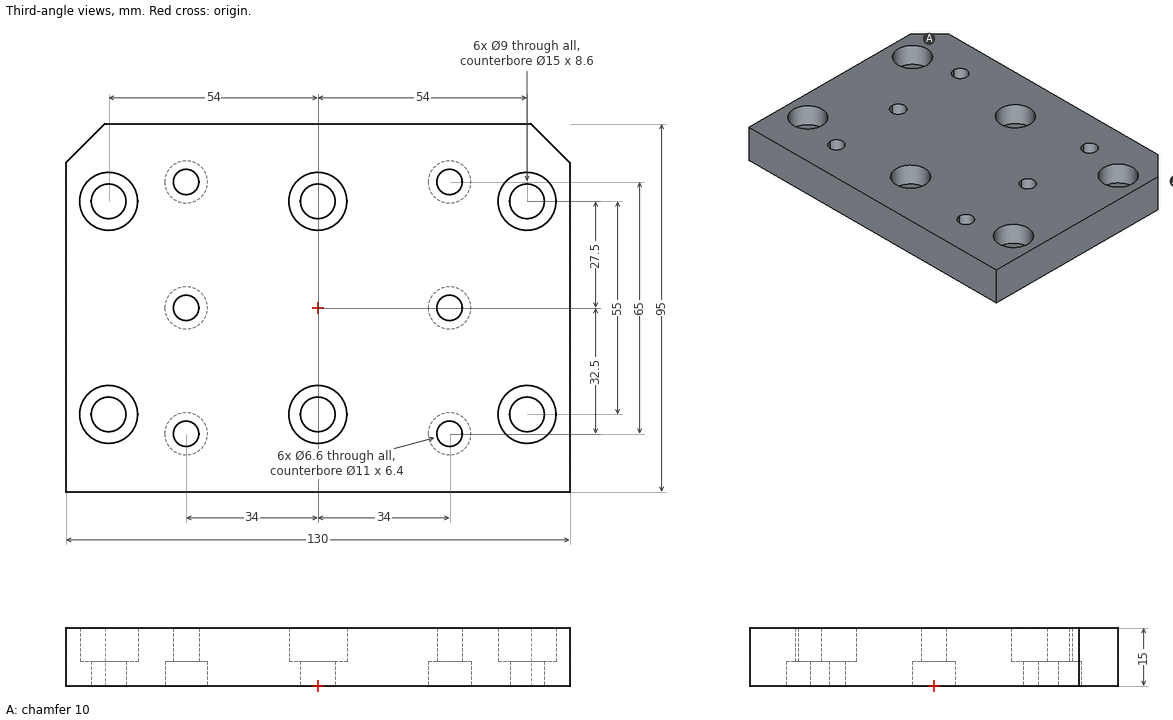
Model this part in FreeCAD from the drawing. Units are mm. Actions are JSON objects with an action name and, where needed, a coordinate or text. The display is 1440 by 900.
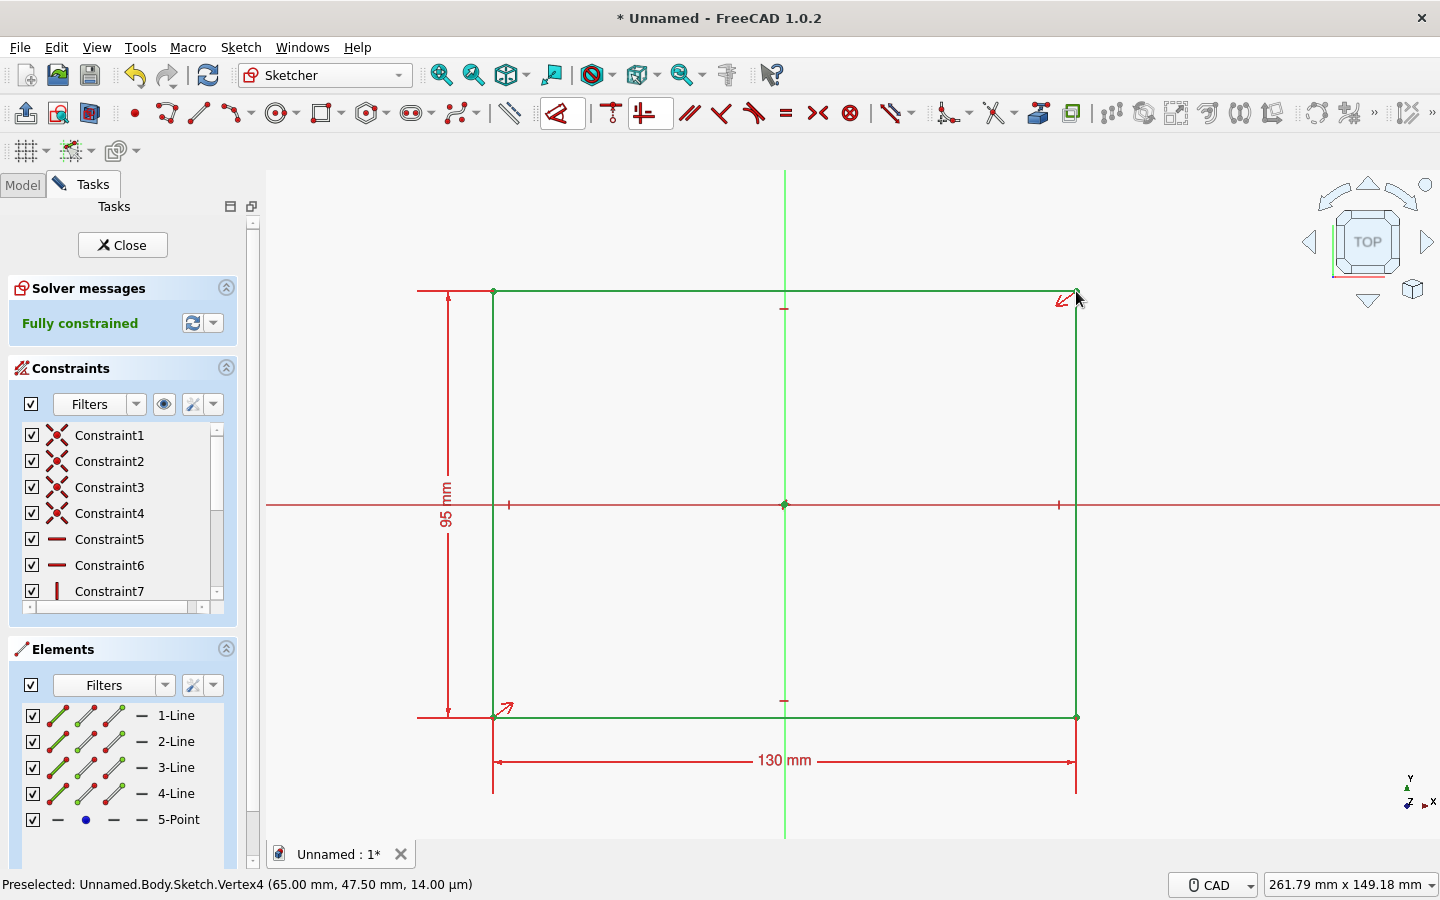
{"action": "left_click", "coordinate": [123, 245]}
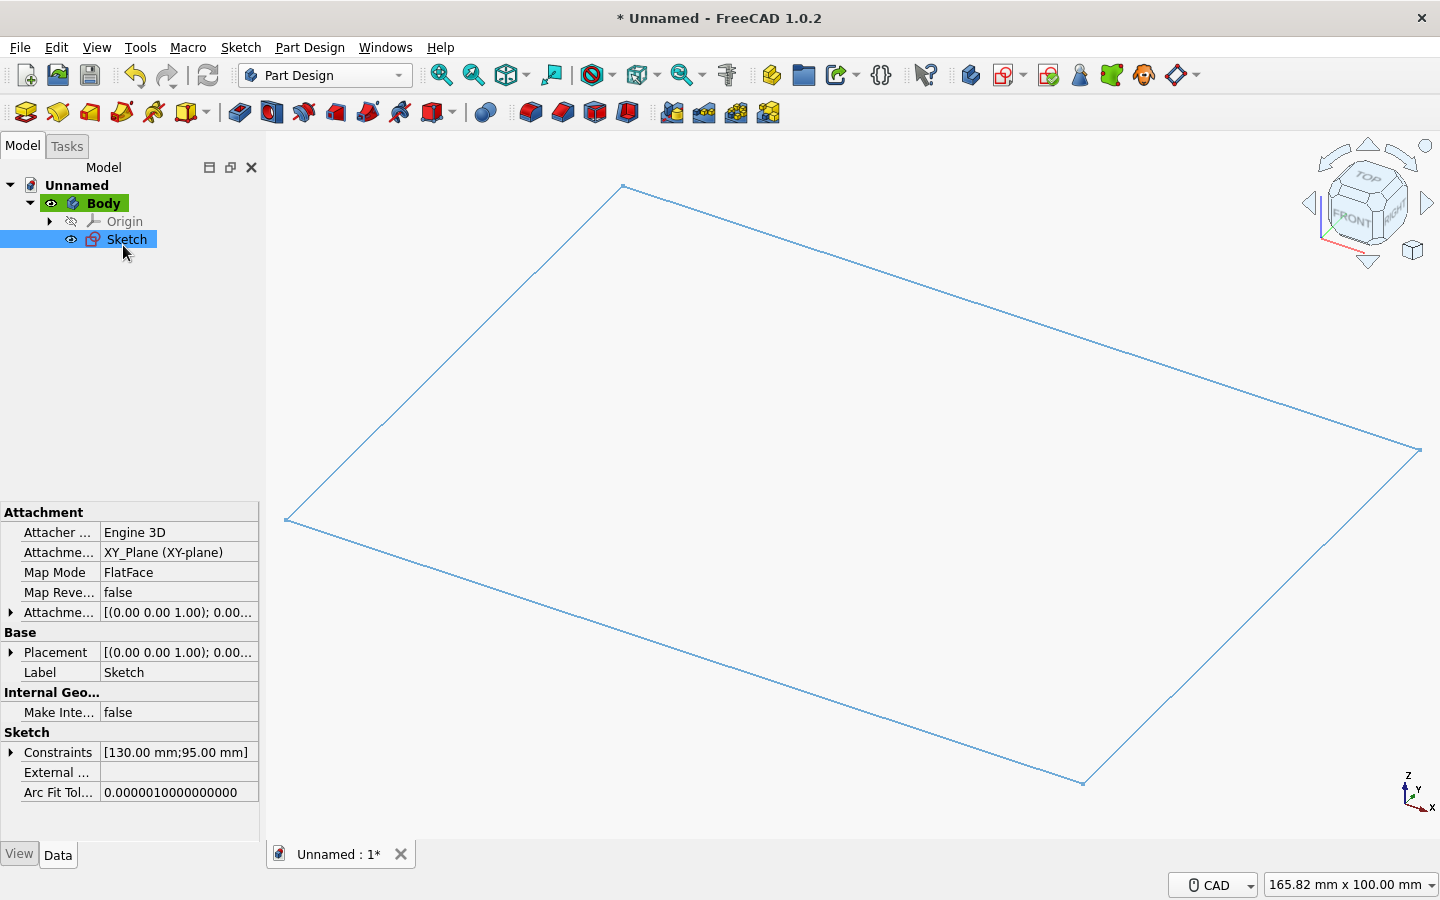
{"action": "left_click", "coordinate": [26, 112]}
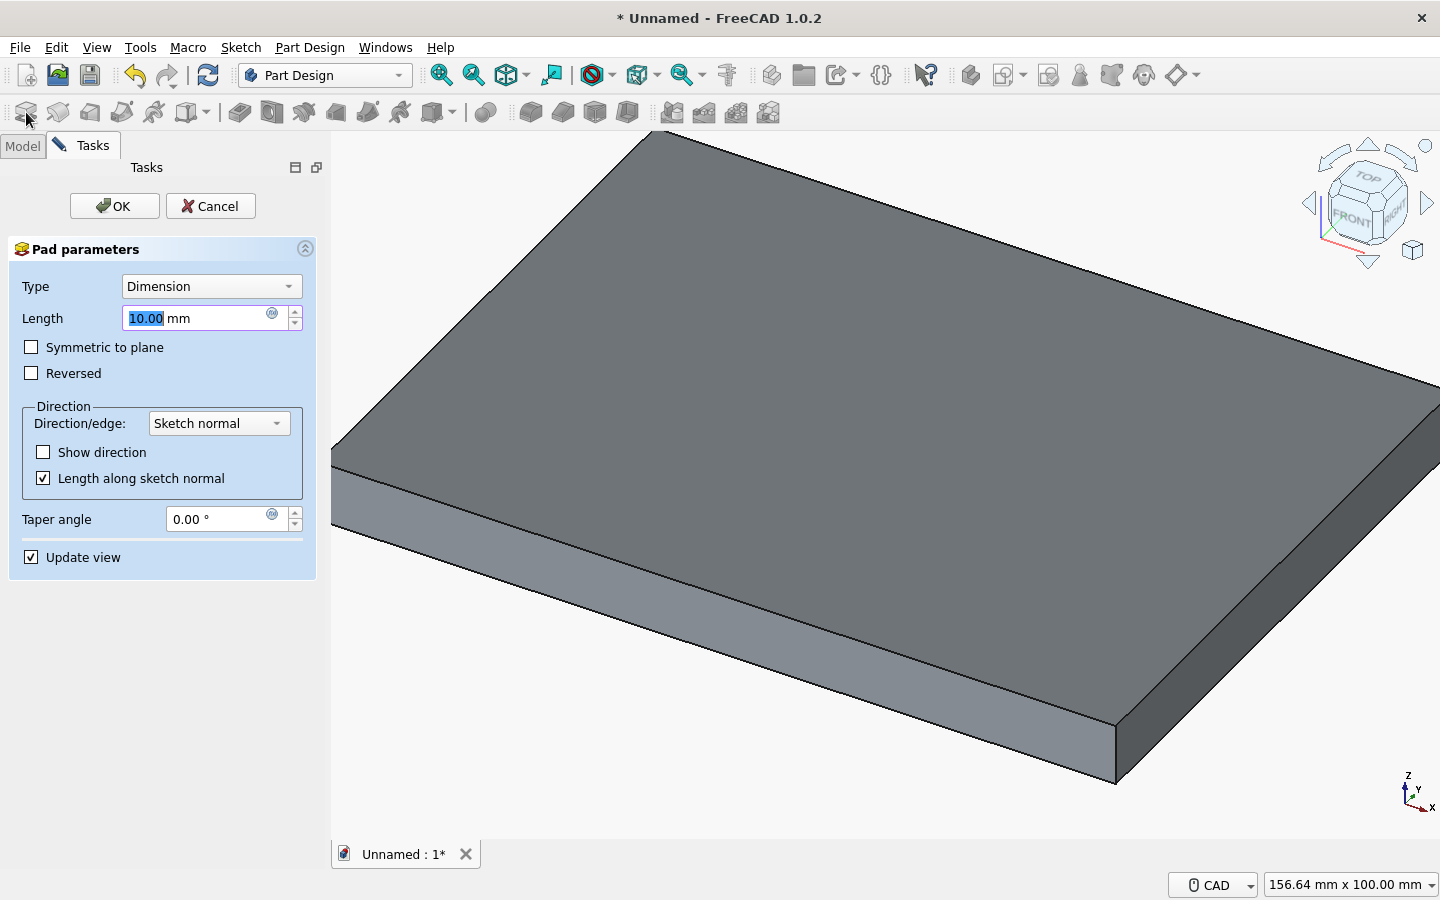
{"action": "type", "text": "15"}
{"action": "key", "text": "Tab"}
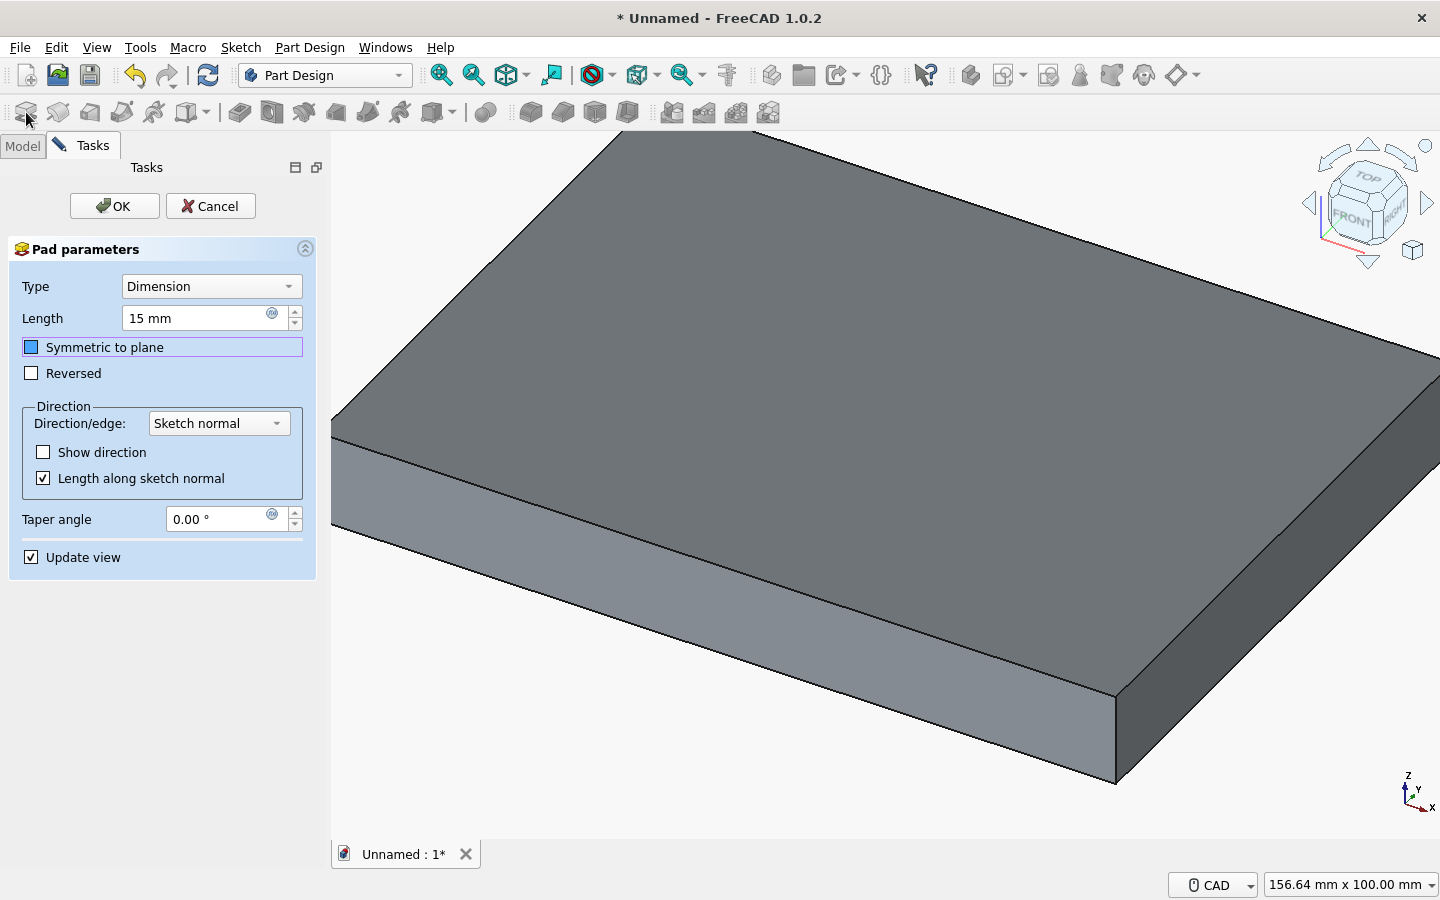
{"action": "left_click", "coordinate": [115, 206]}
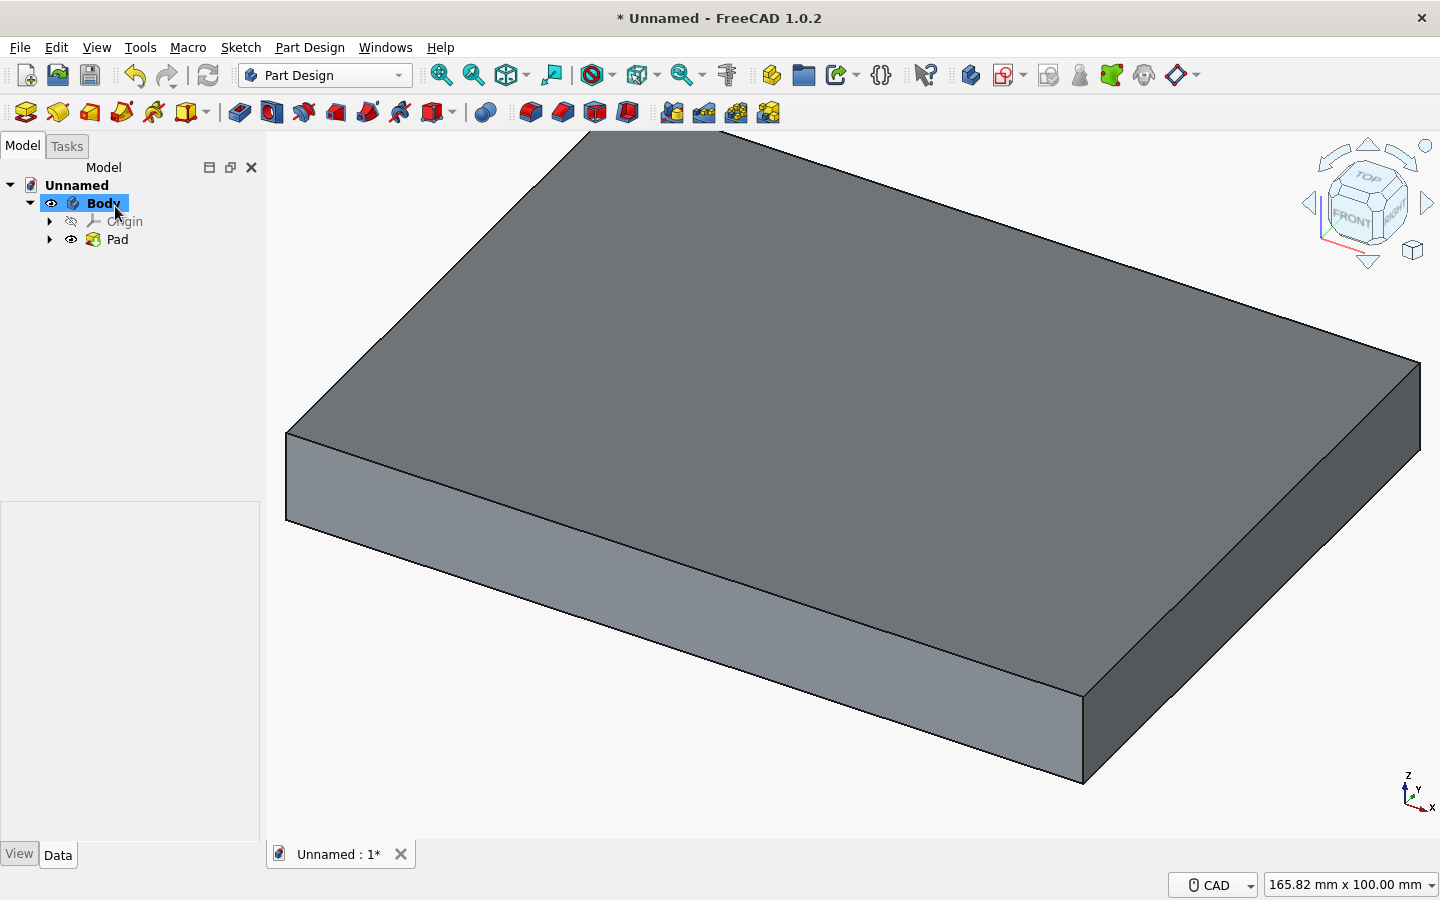
{"action": "key", "text": "v f"}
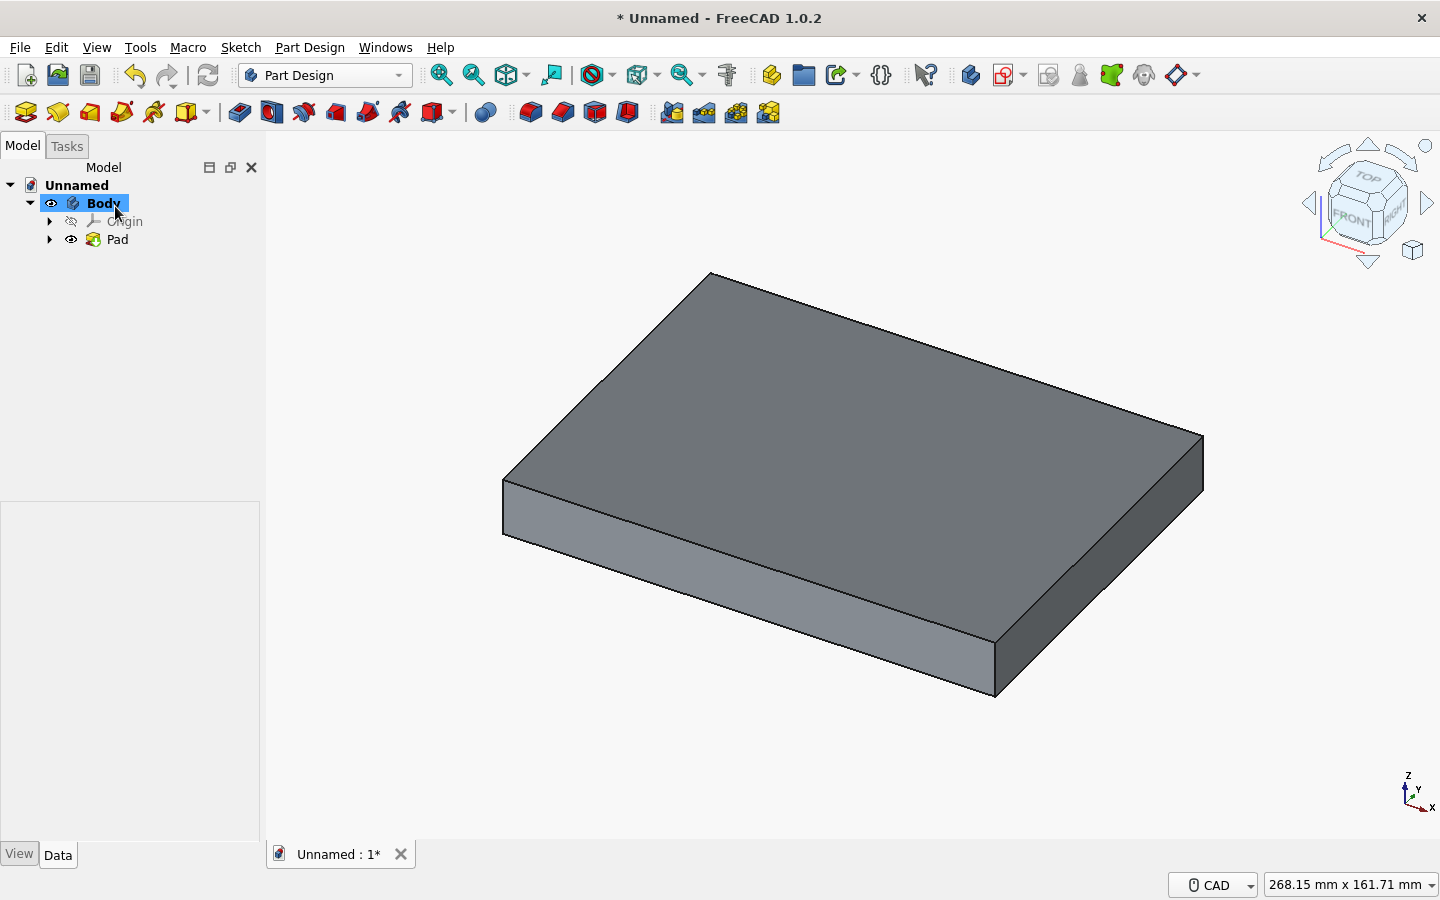
{"action": "left_click", "coordinate": [853, 457]}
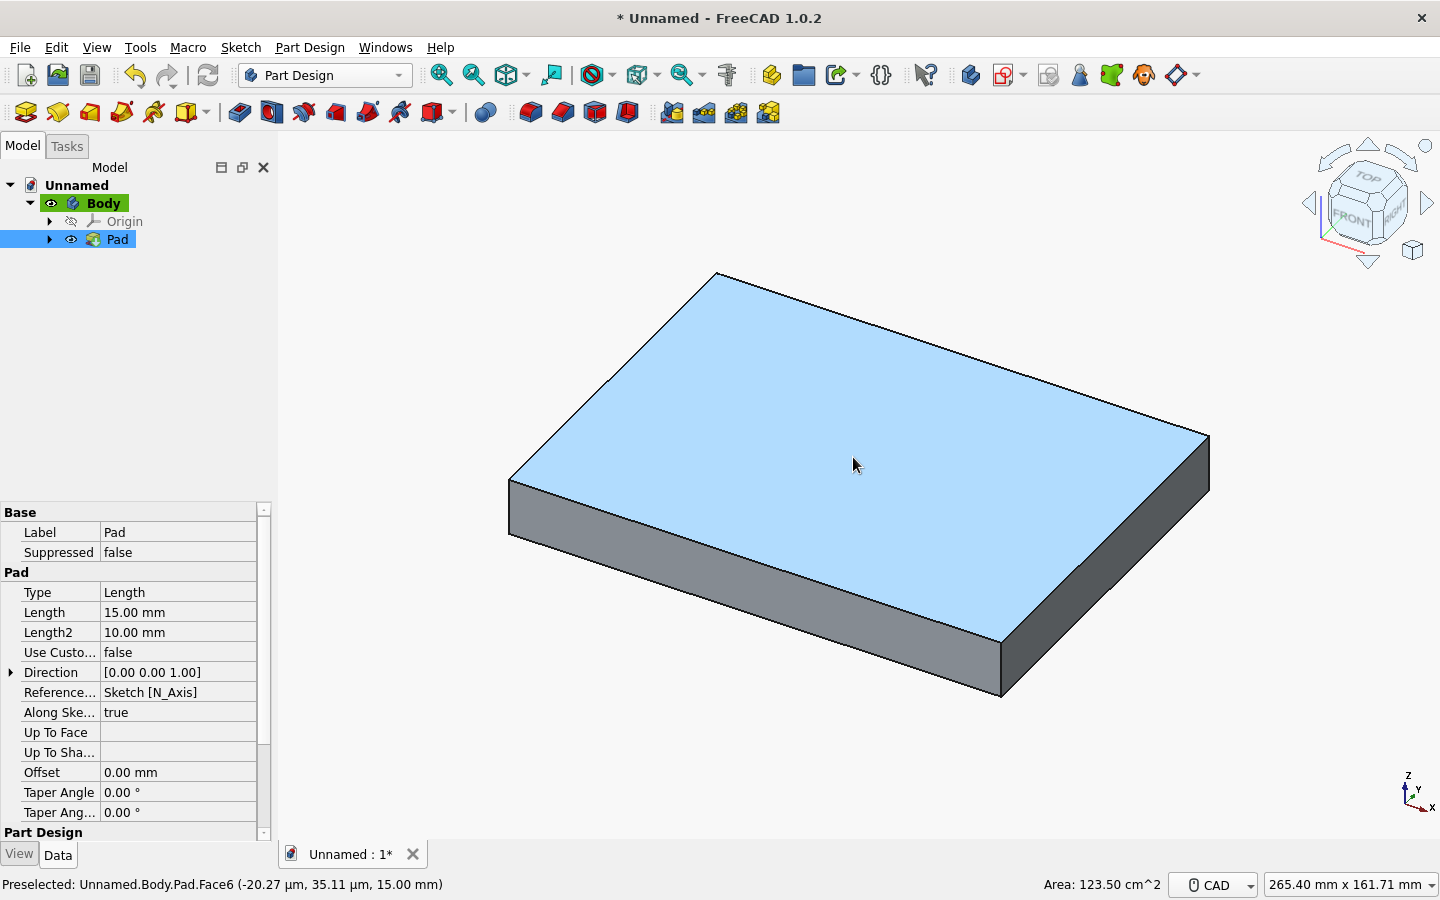
{"action": "left_click", "coordinate": [1004, 76]}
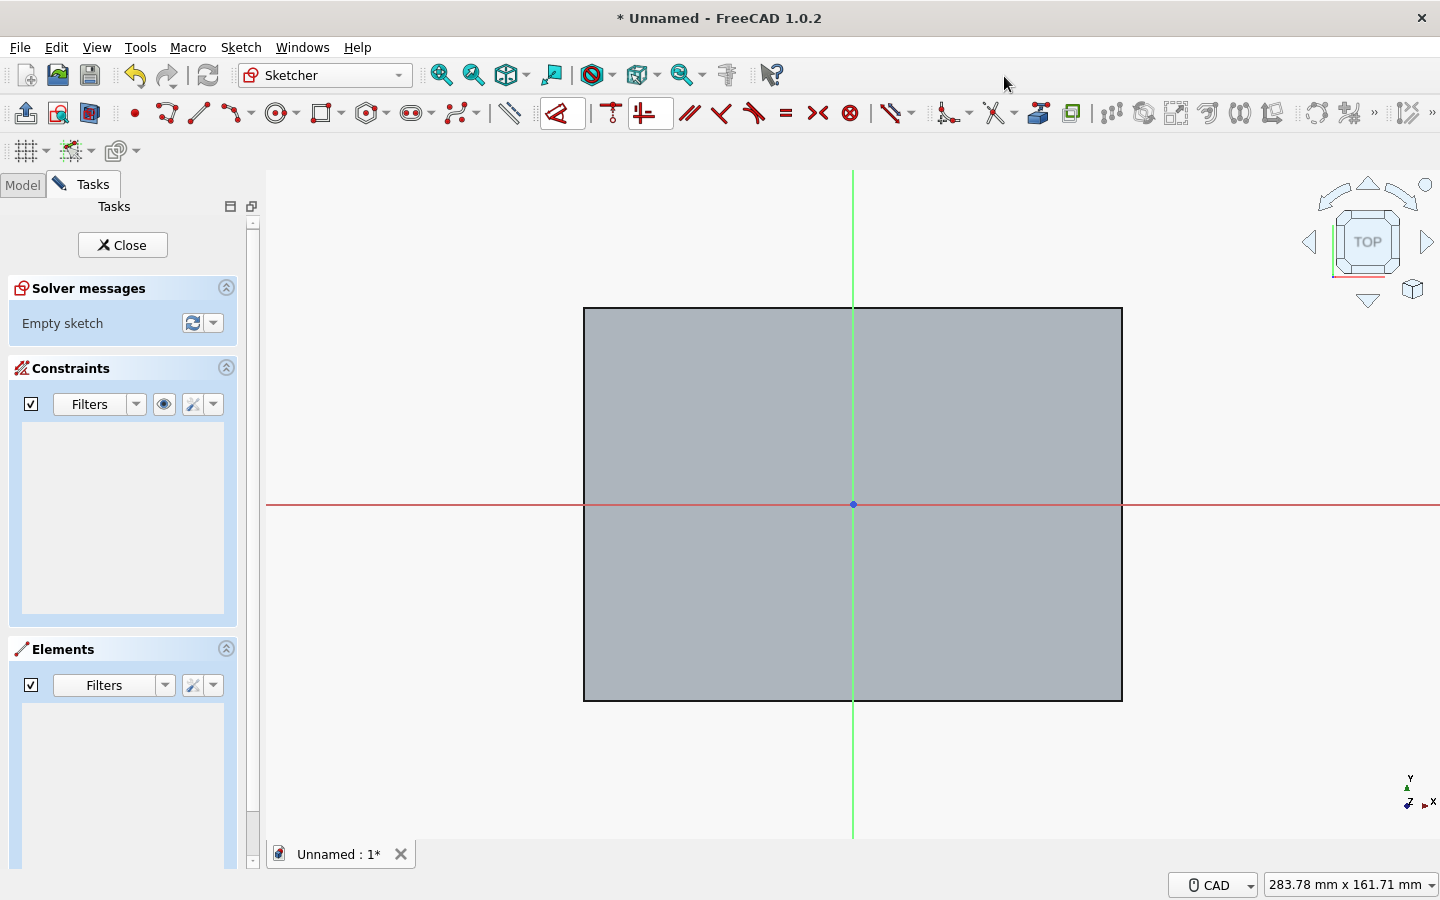
{"action": "scroll", "coordinate": [992, 504], "scroll_direction": "up", "scroll_amount": 2}